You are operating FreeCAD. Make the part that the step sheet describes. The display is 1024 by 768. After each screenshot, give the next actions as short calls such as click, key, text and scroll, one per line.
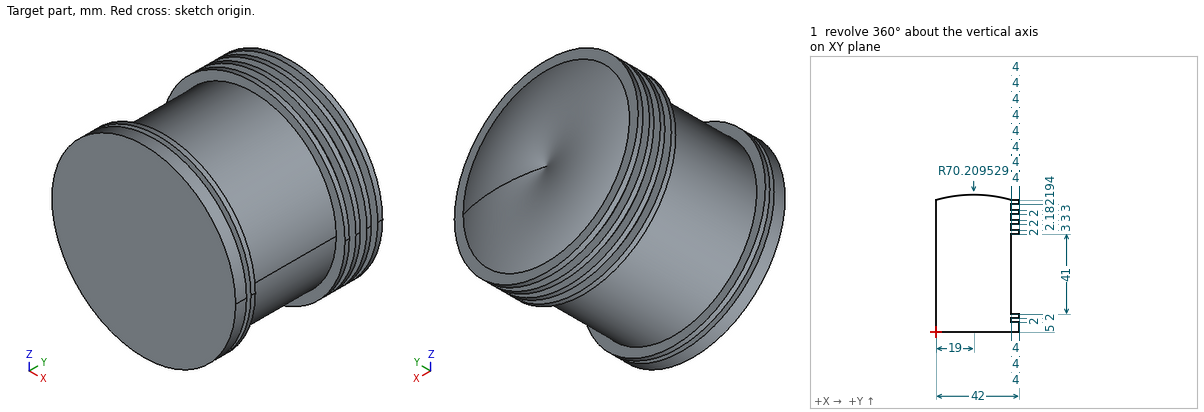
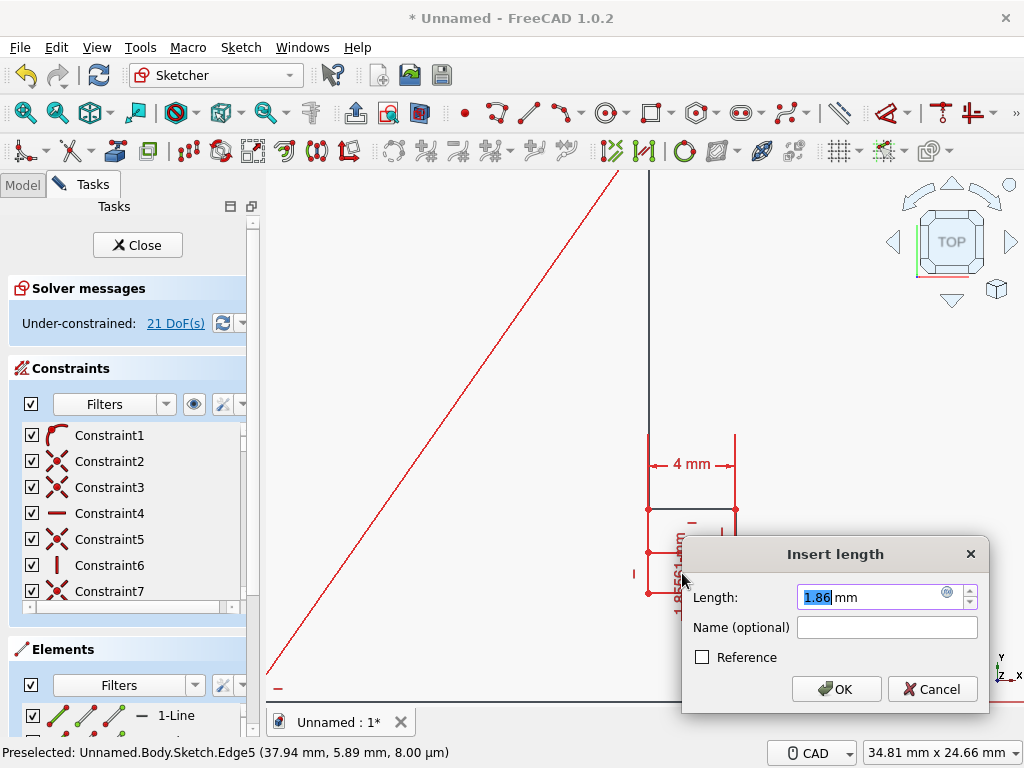
text(2)
key(Return)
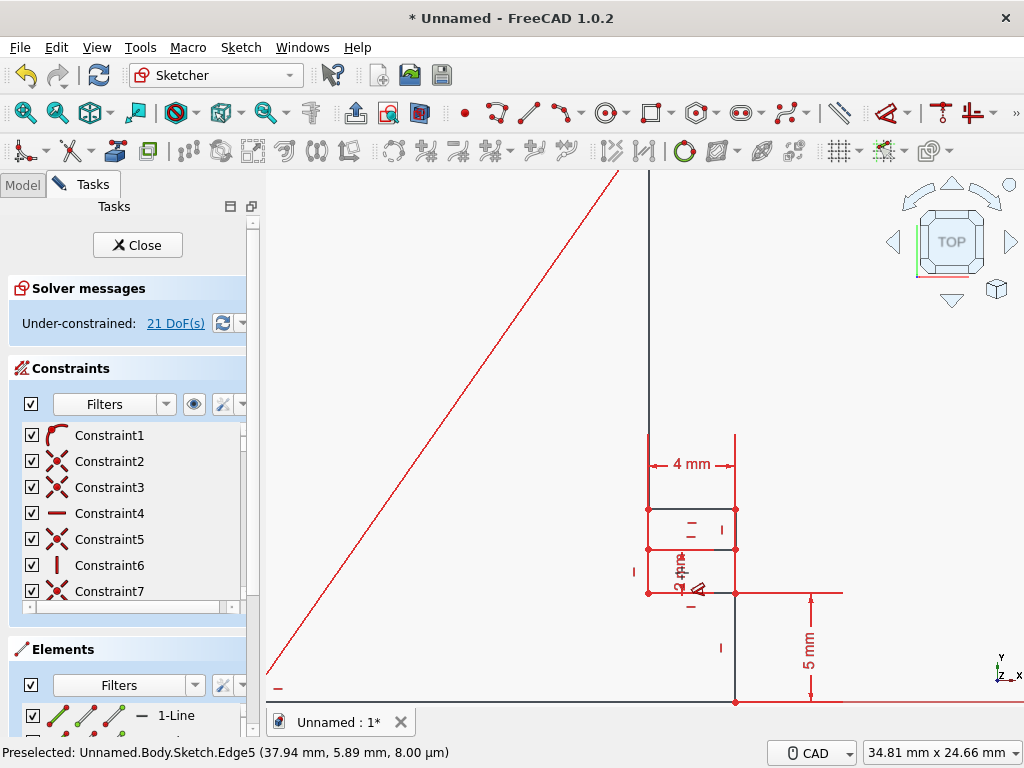
click(674, 550)
click(692, 608)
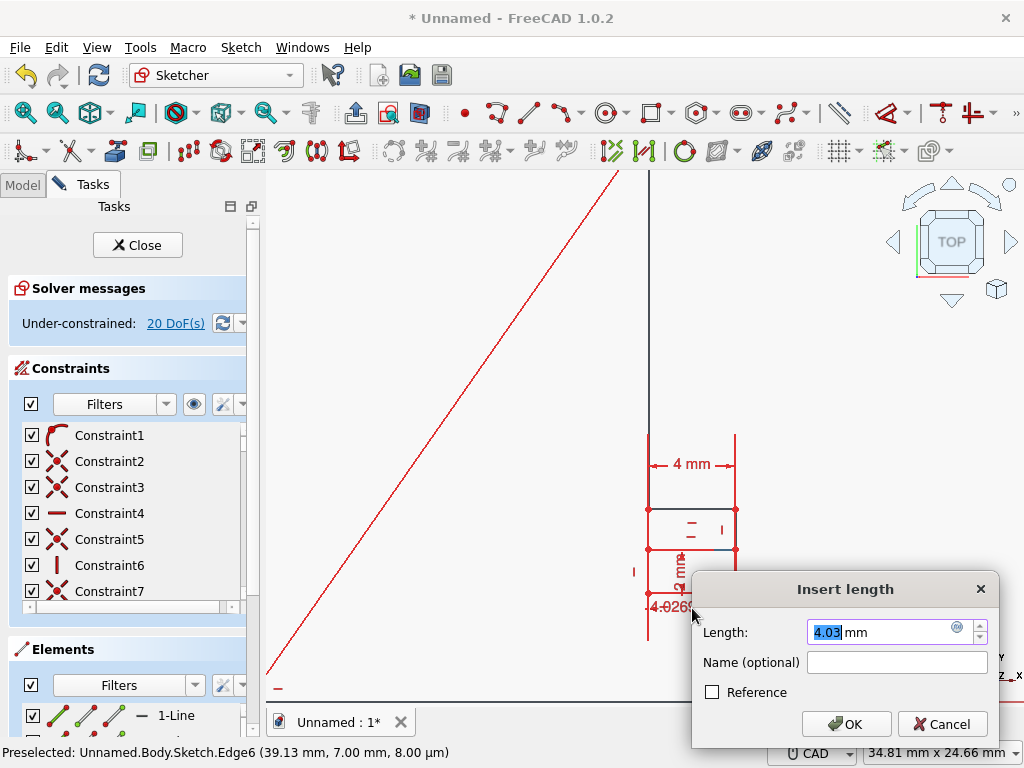
text(4)
key(Return)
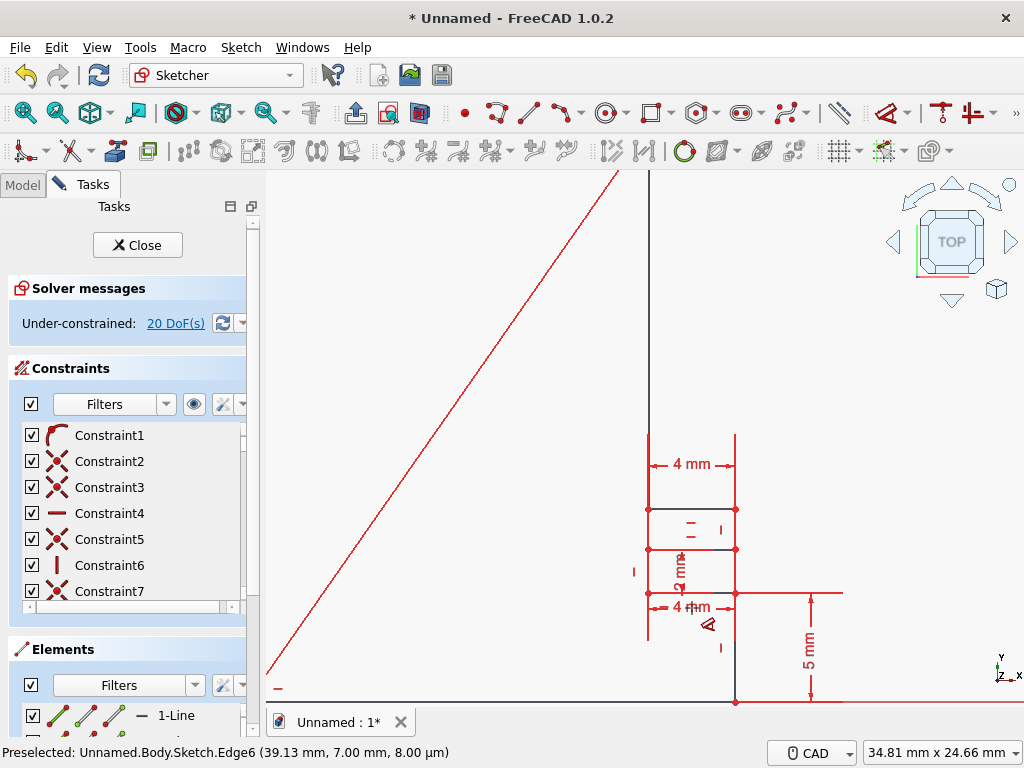
click(735, 538)
click(769, 530)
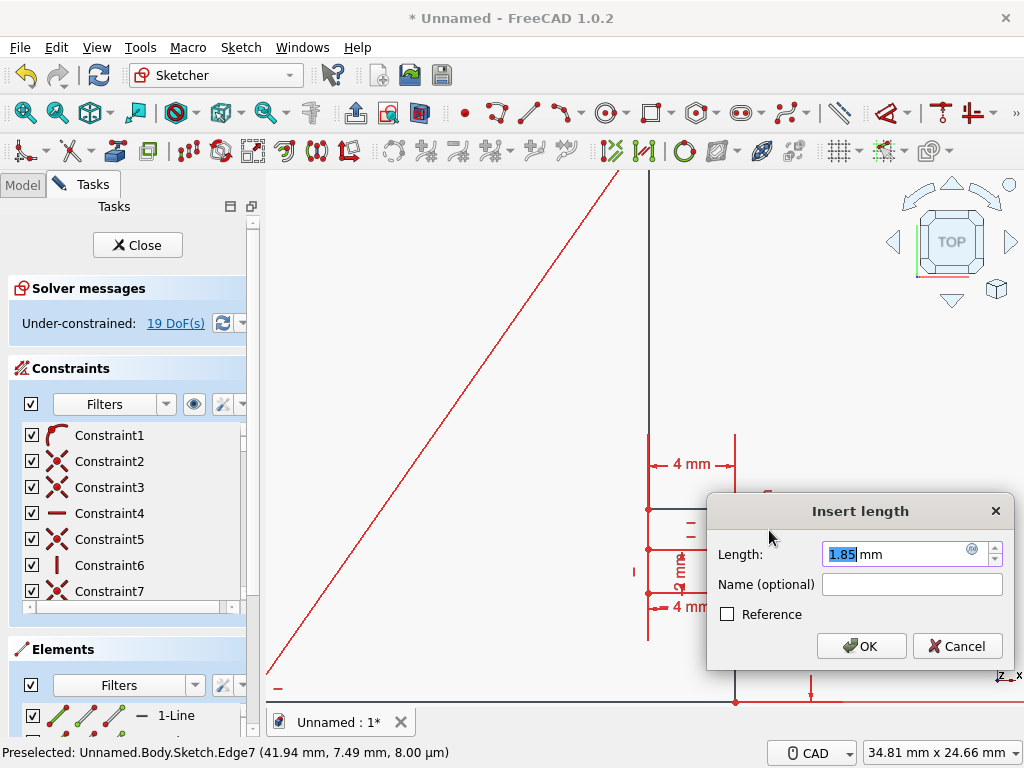
text(2)
key(Return)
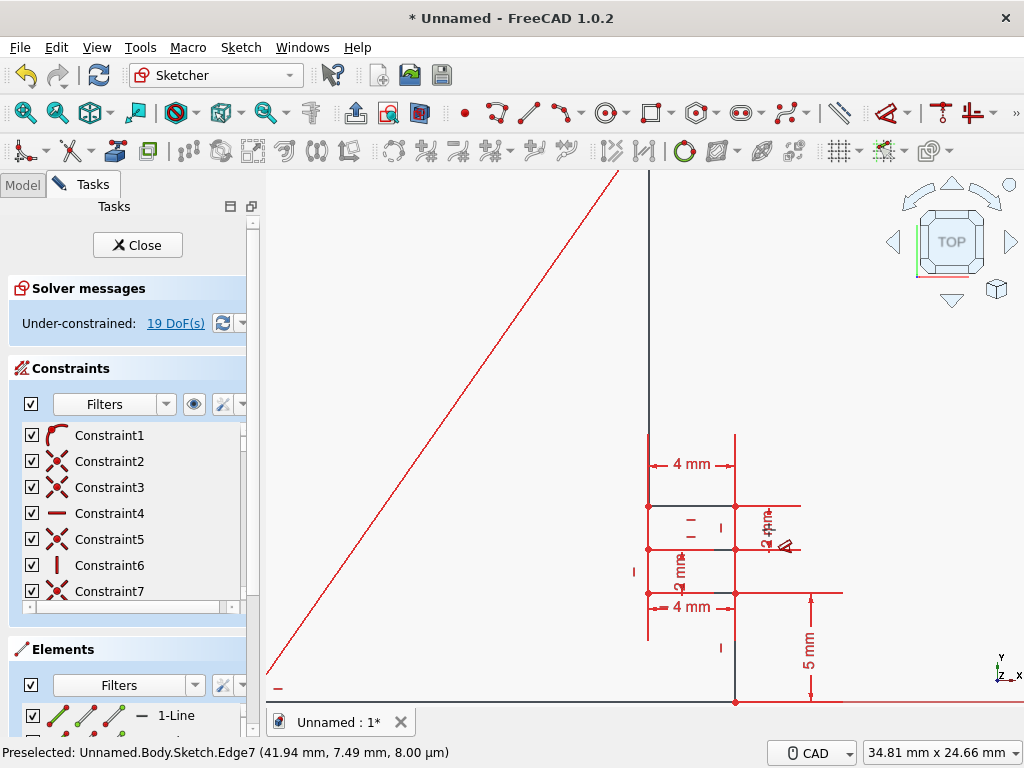
click(709, 506)
click(692, 424)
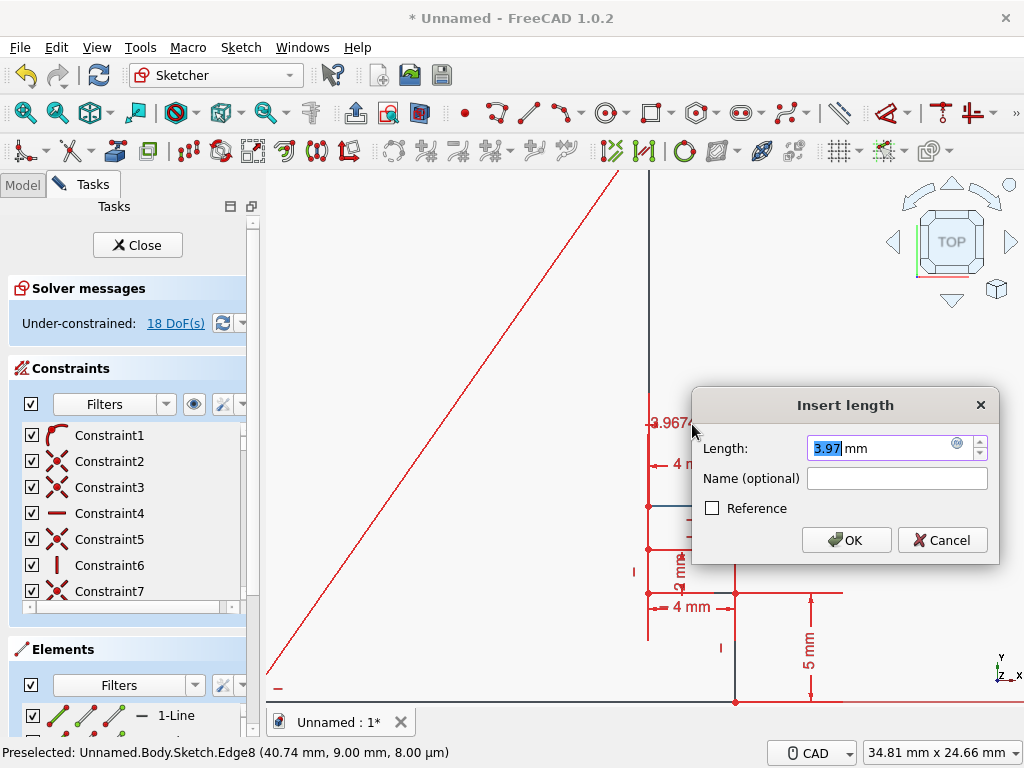
text(4)
key(Return)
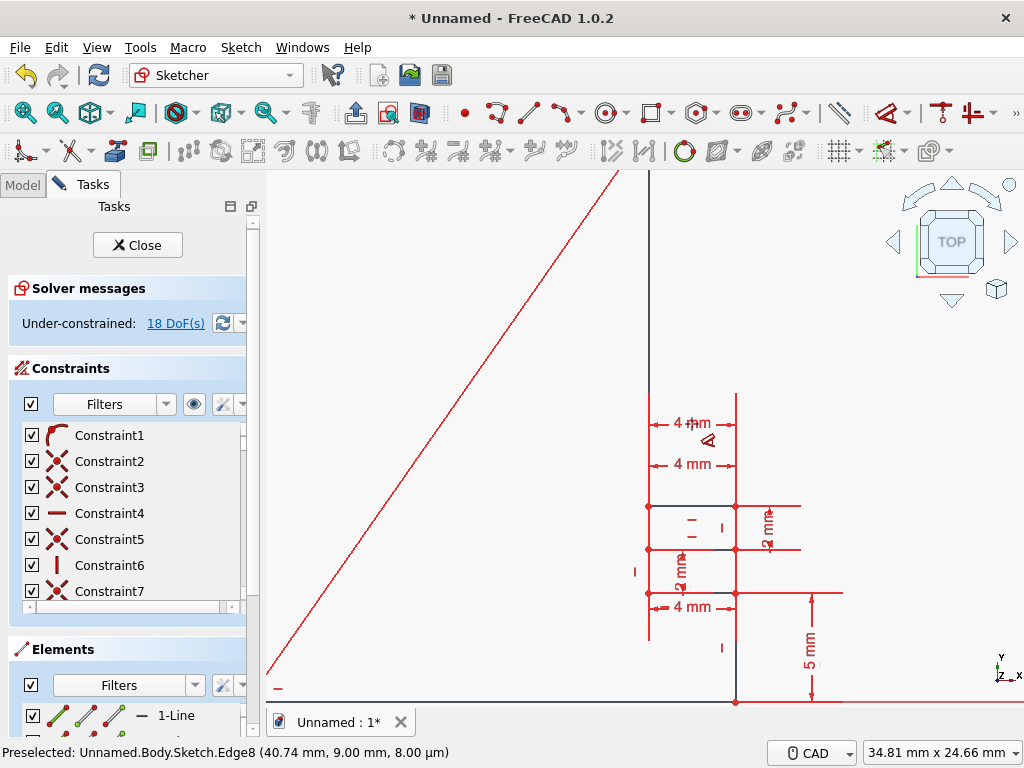
scroll(674, 601, down, 7)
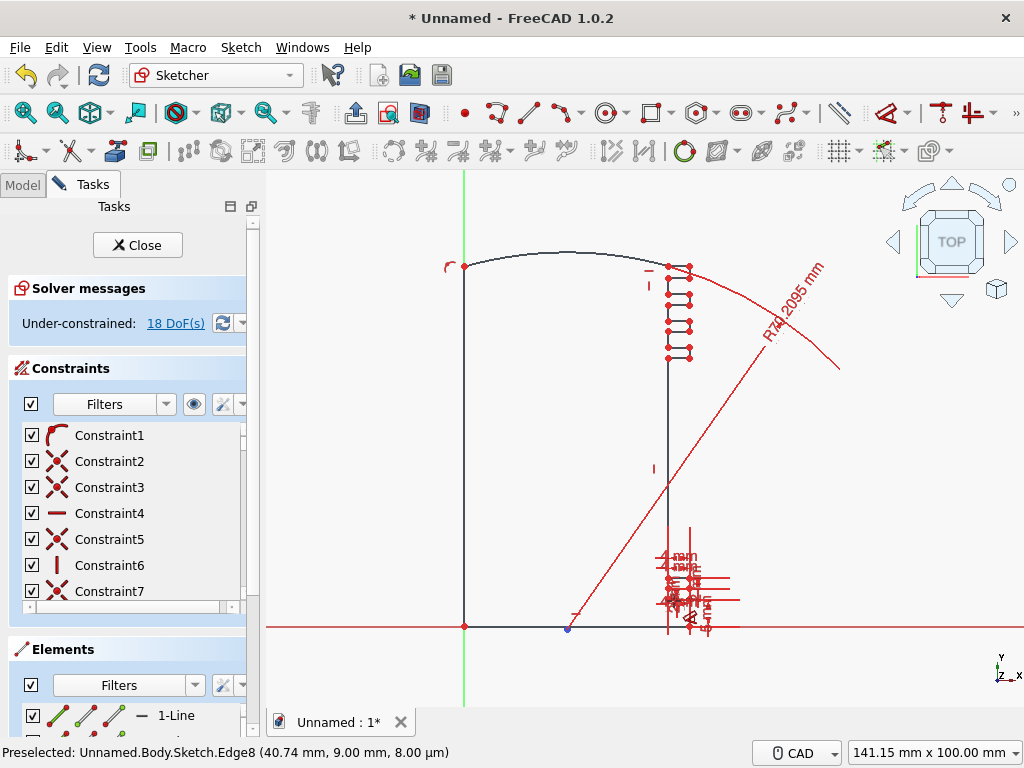
scroll(675, 358, up, 4)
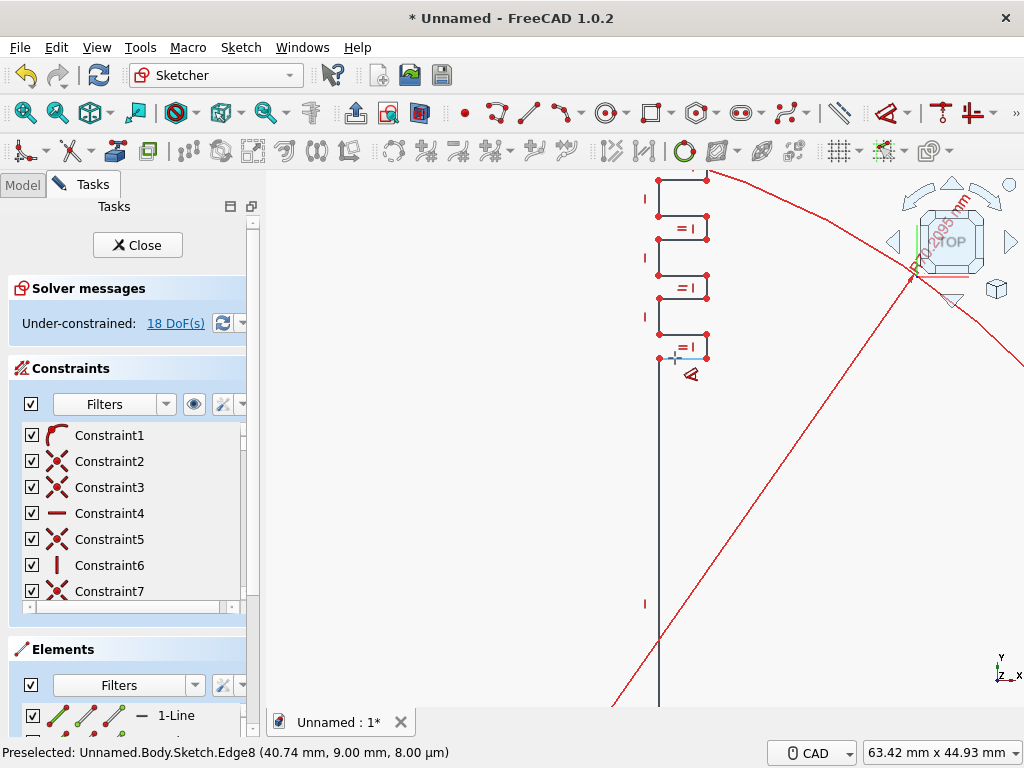
click(673, 359)
click(683, 393)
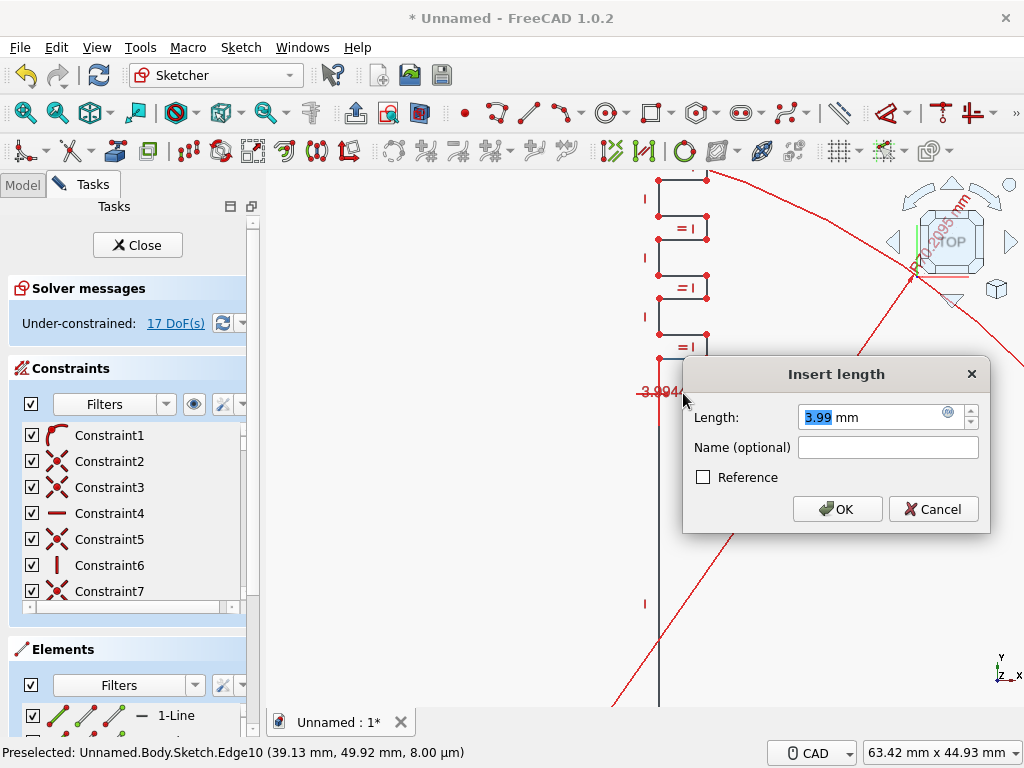
text(4)
key(Return)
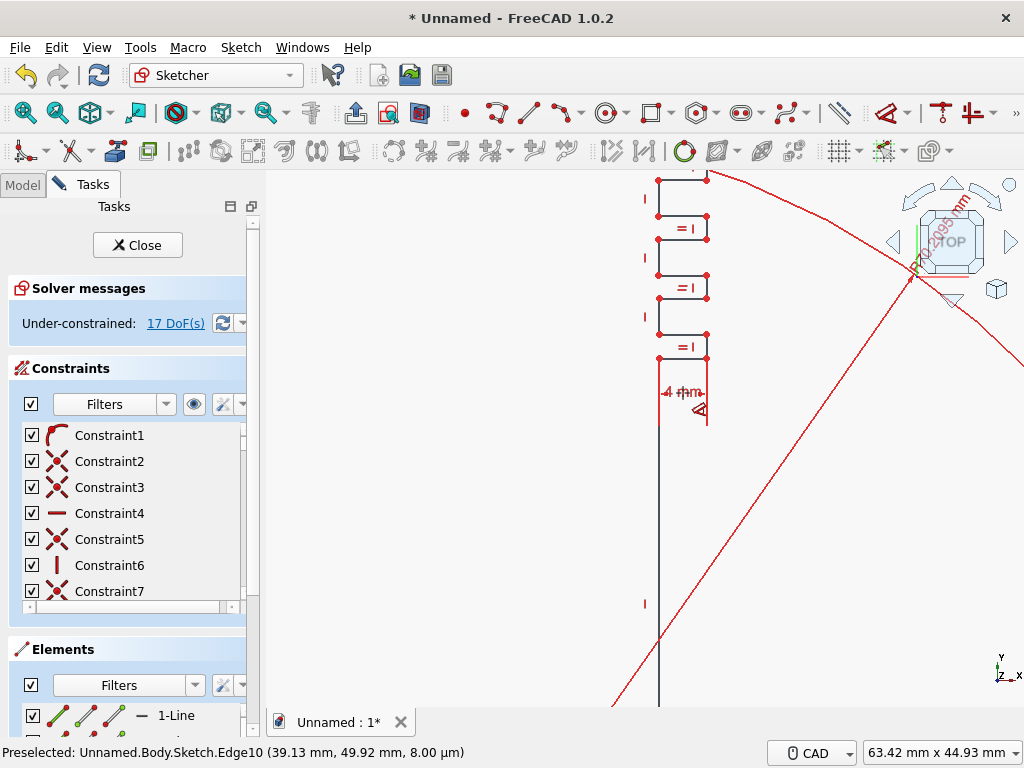
scroll(707, 349, up, 3)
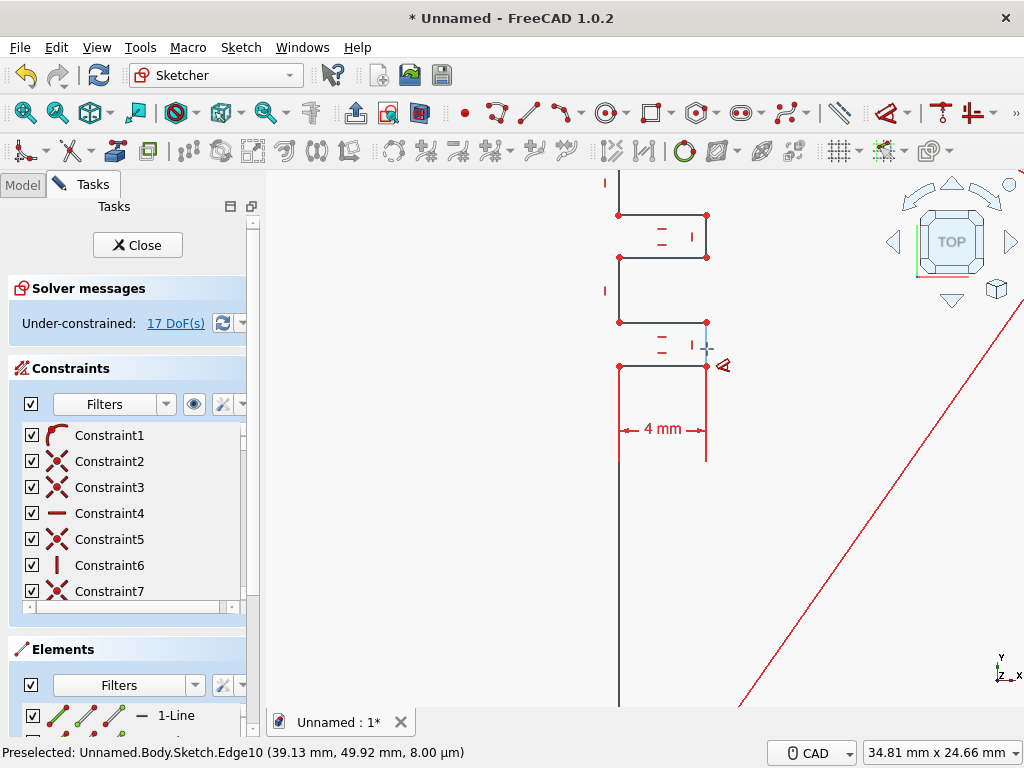
click(706, 349)
click(740, 345)